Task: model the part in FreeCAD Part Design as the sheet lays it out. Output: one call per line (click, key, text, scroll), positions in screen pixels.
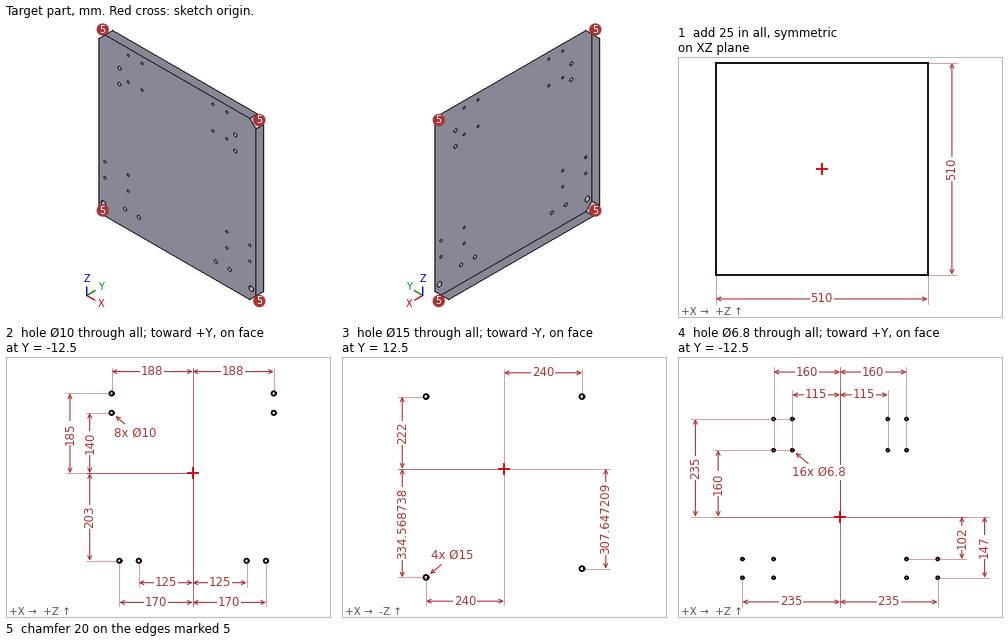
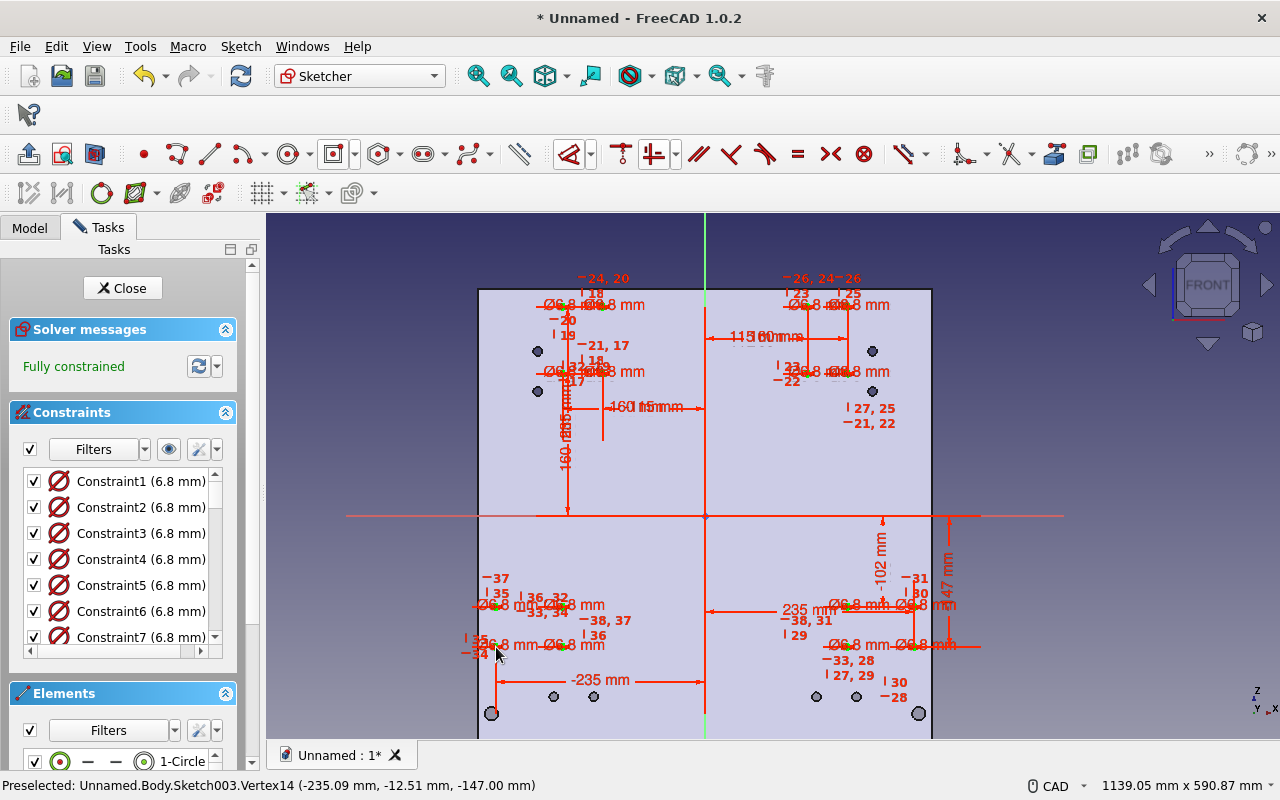
click(123, 288)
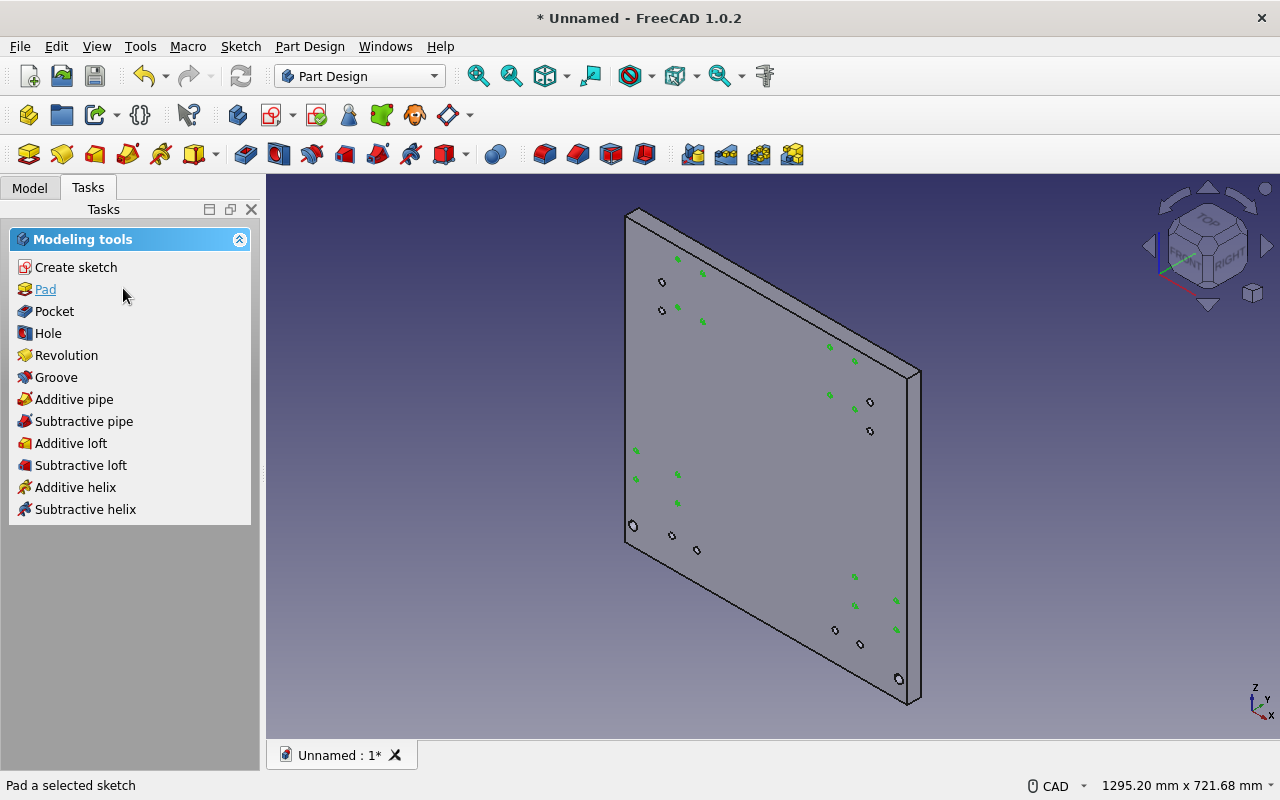
click(279, 154)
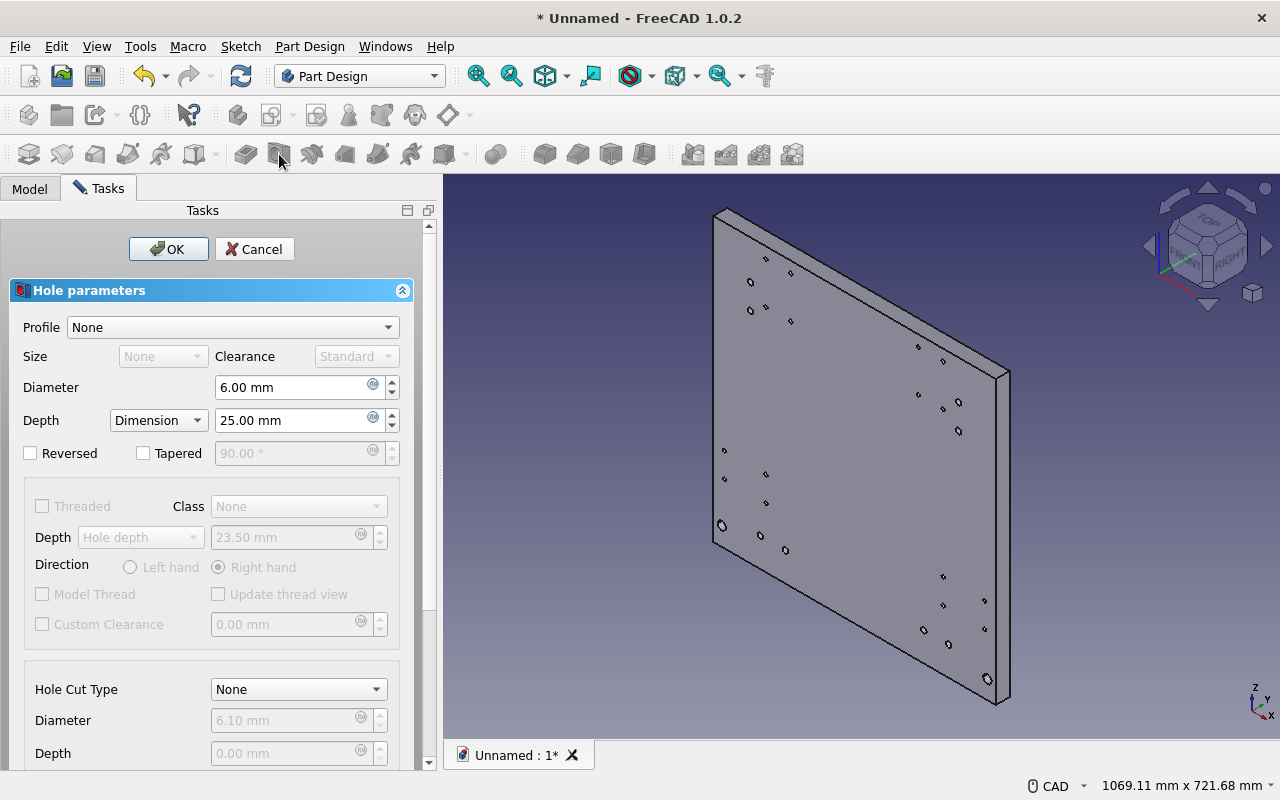
triple_click(300, 388)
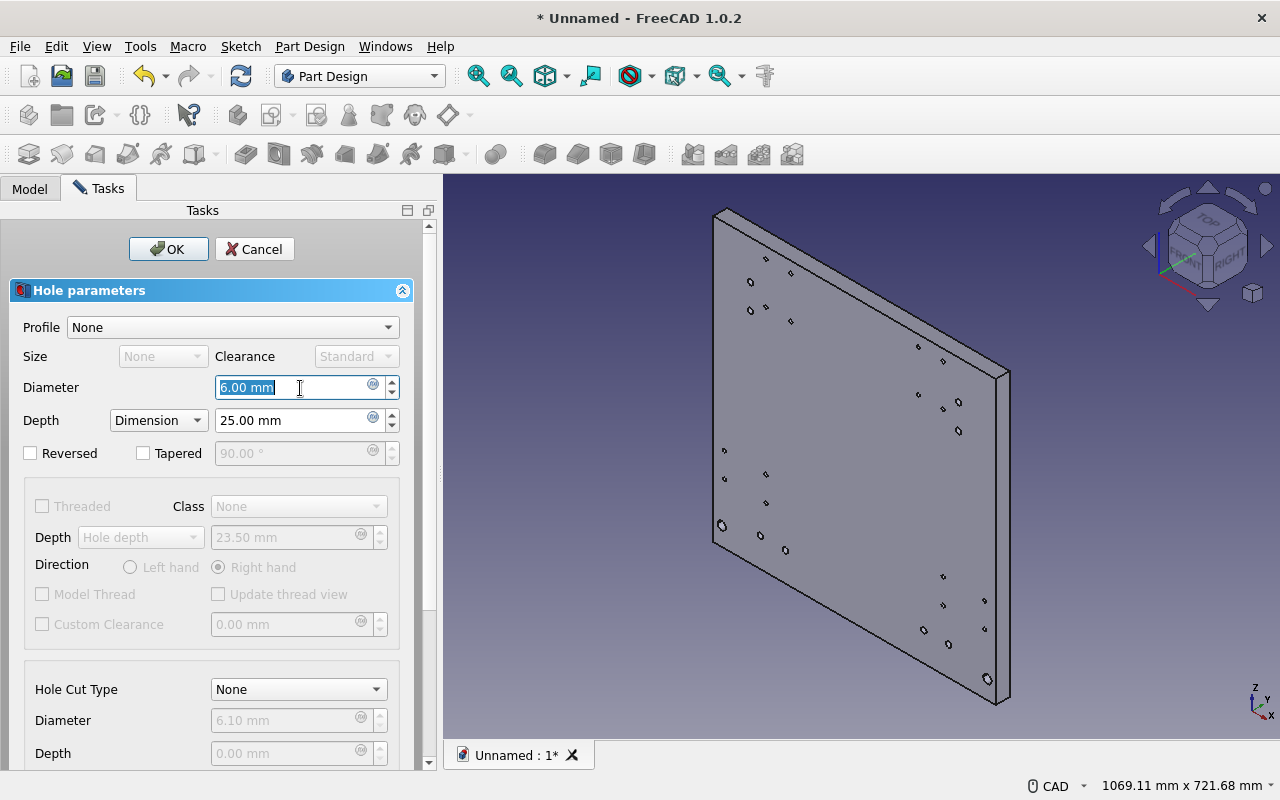
text(6.8)
key(Tab)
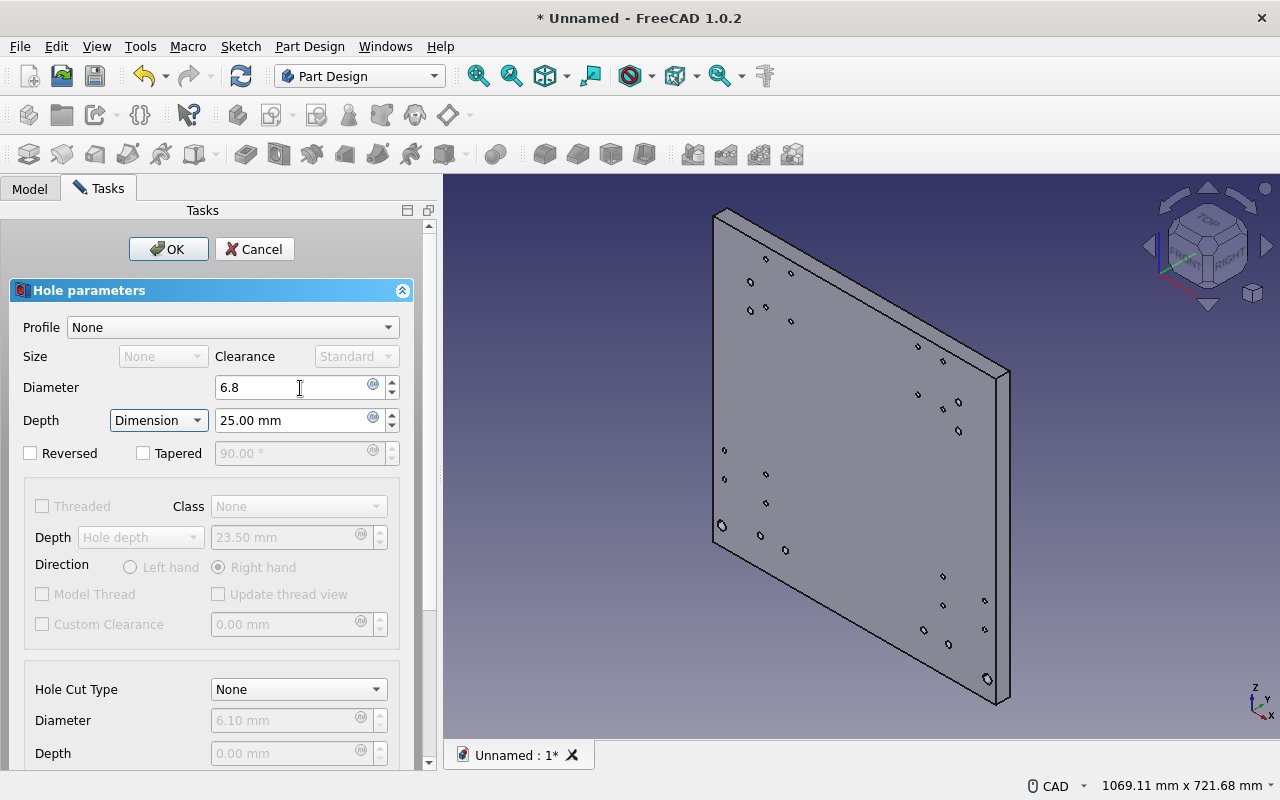
click(160, 420)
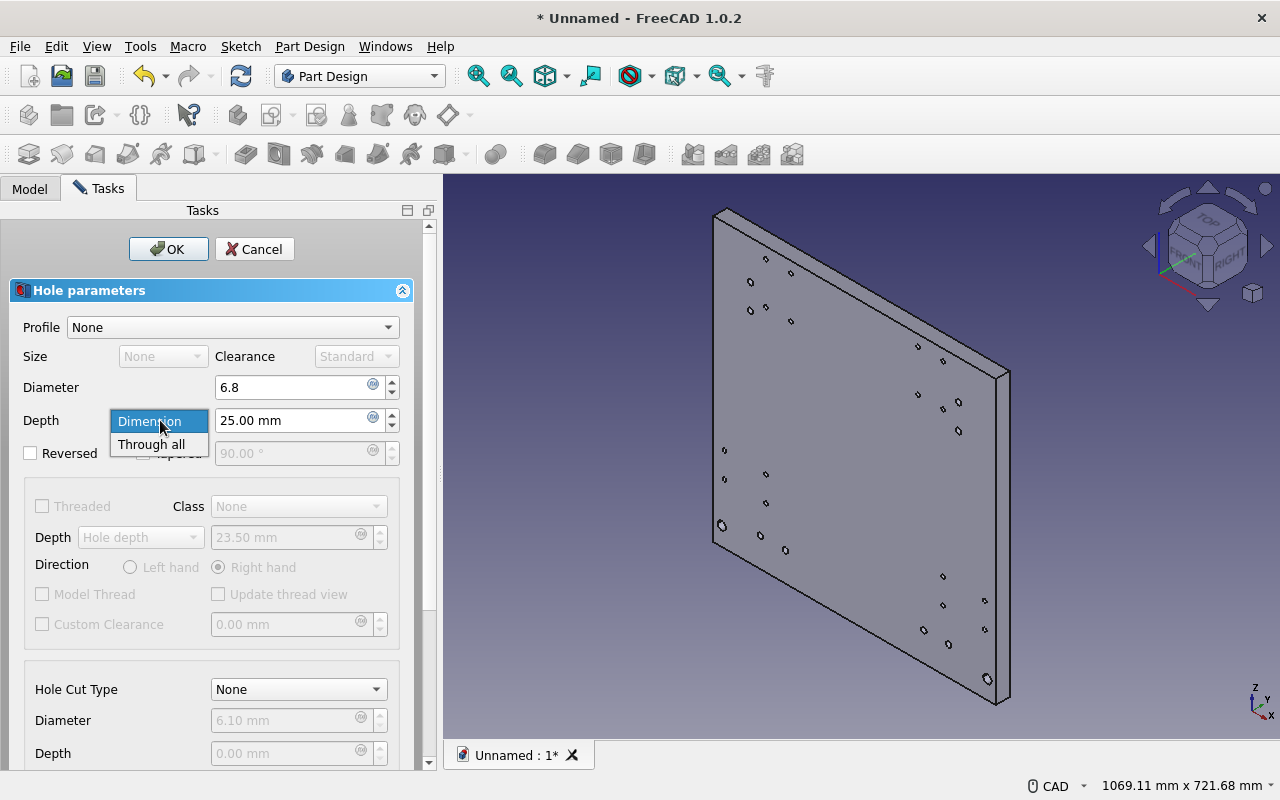
click(158, 444)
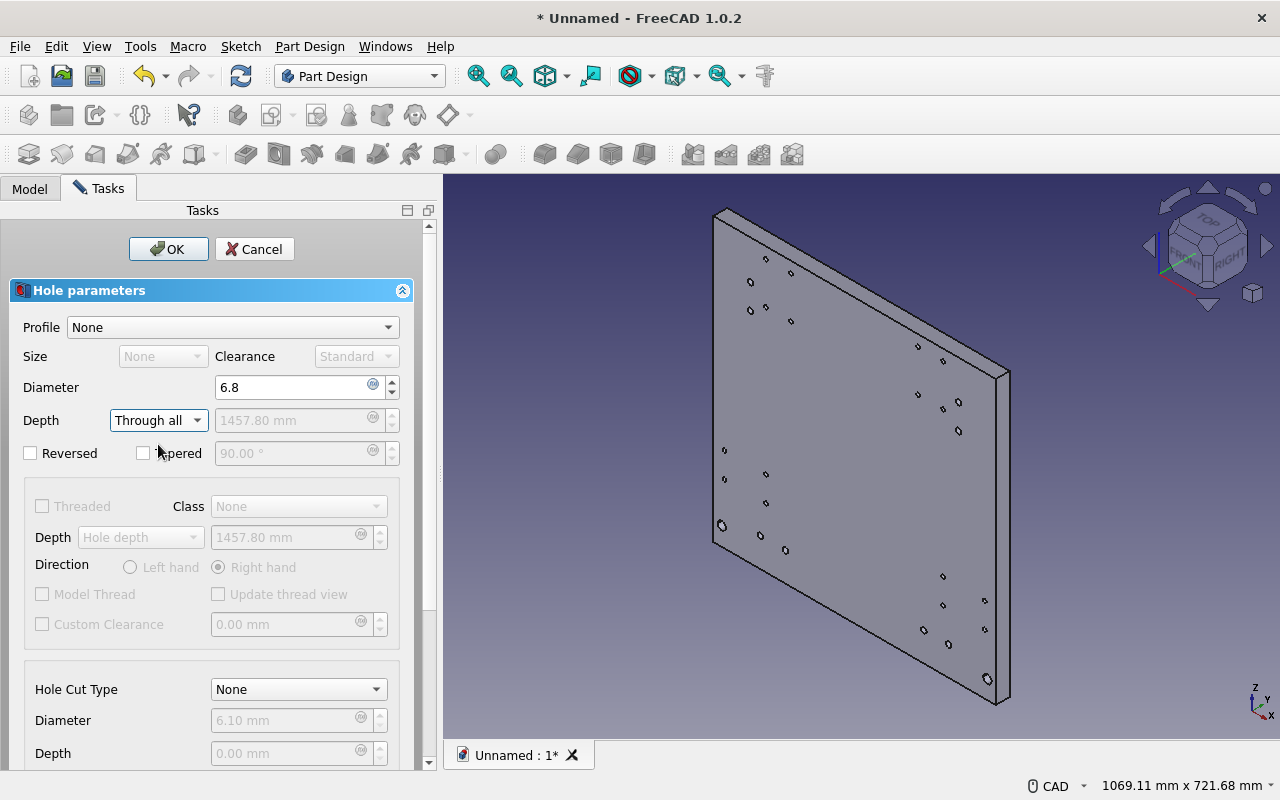
click(169, 249)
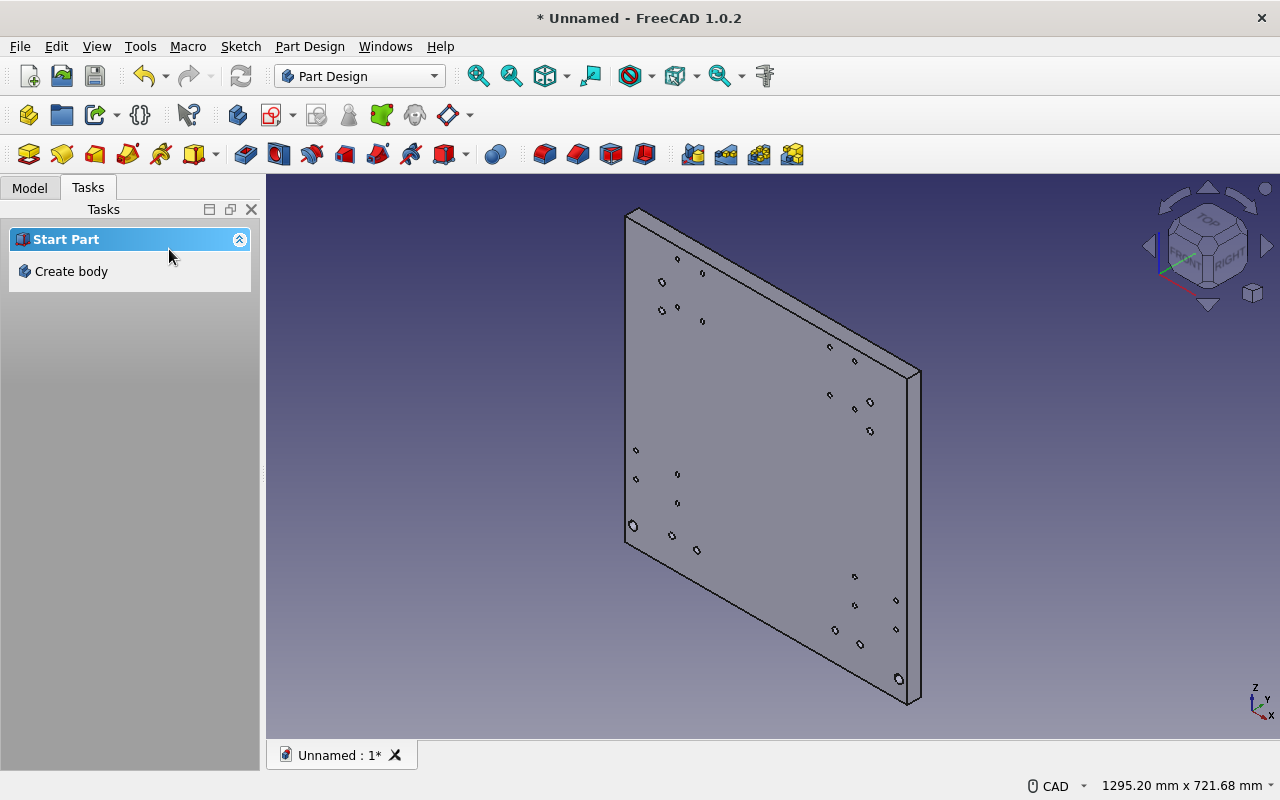
click(914, 374)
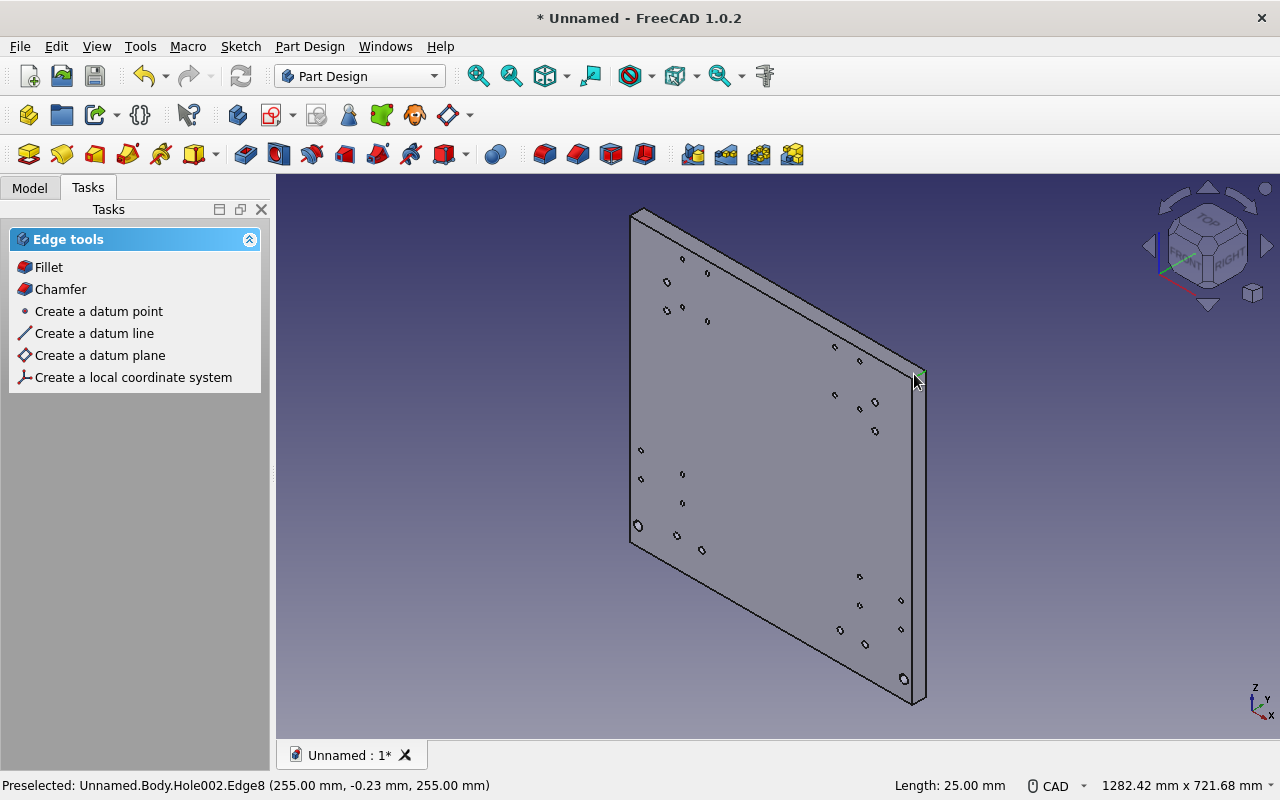
scroll(637, 537, up, 4)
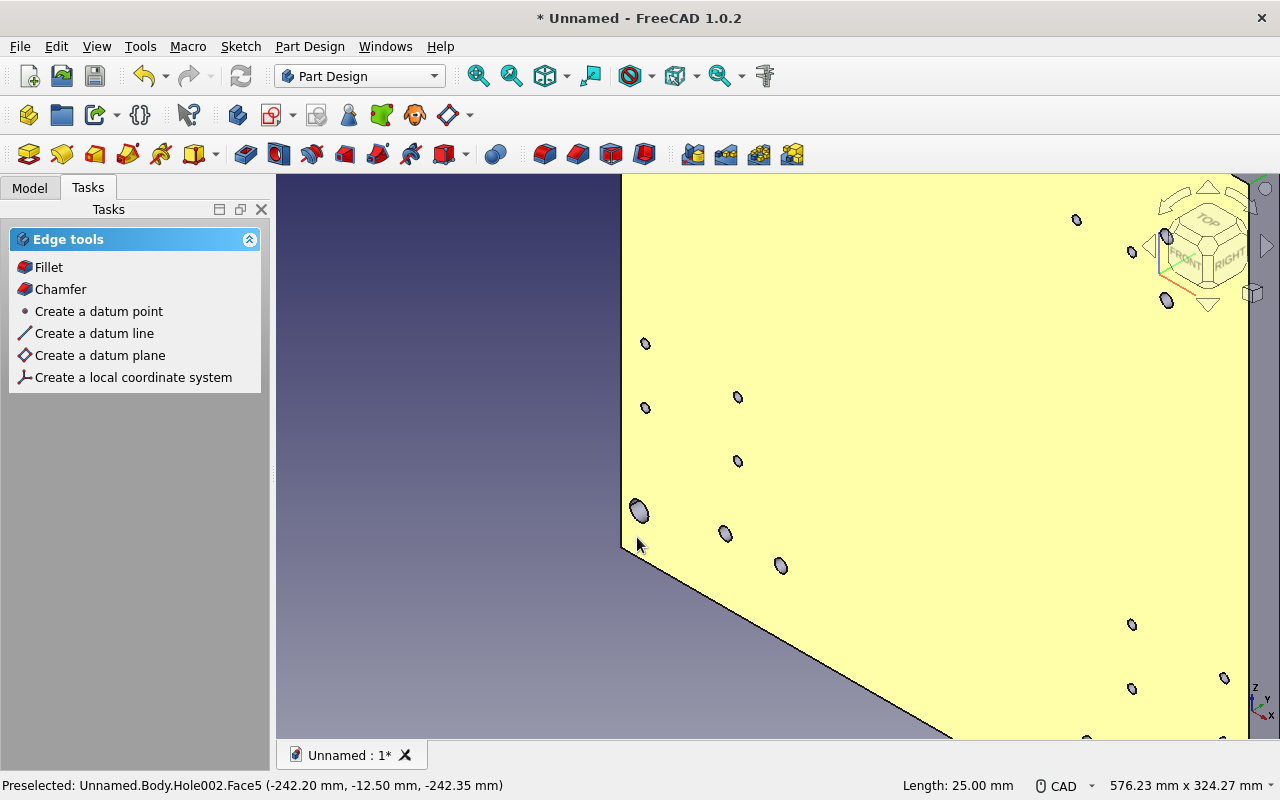
click(479, 76)